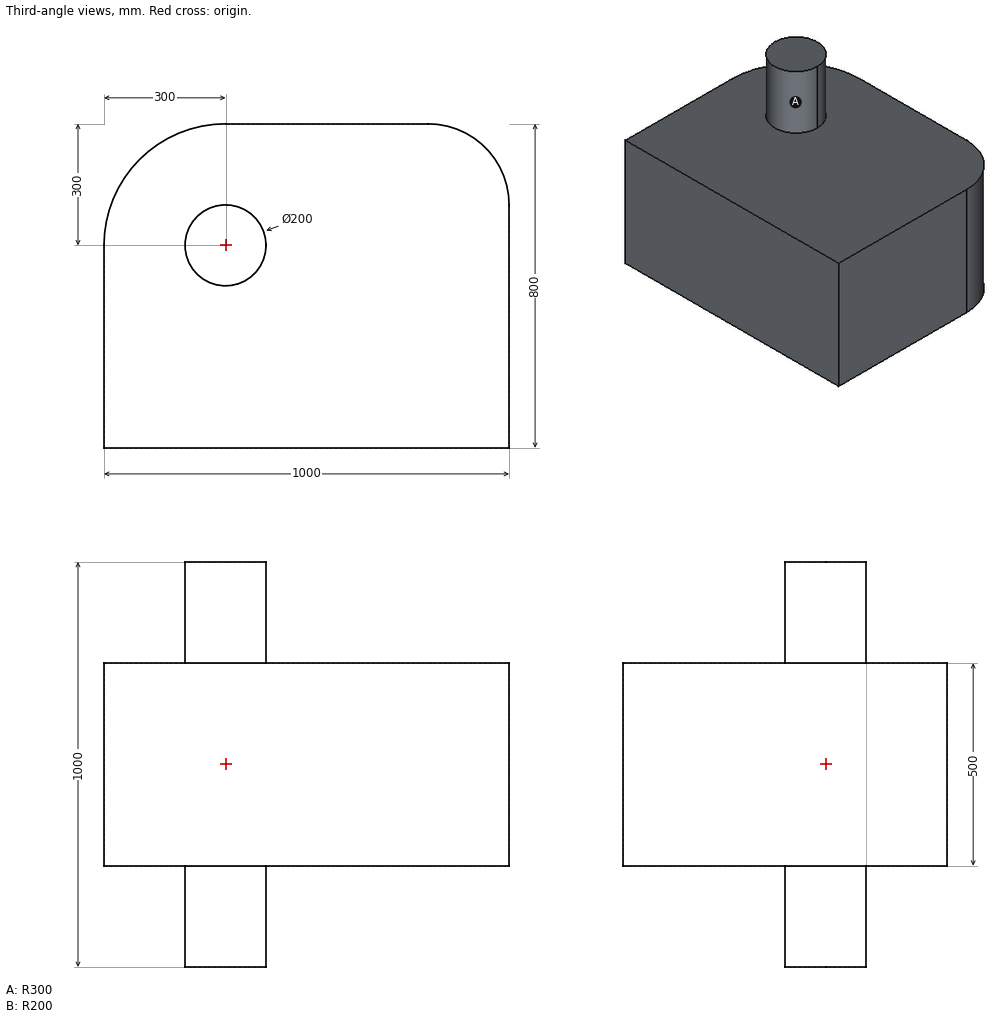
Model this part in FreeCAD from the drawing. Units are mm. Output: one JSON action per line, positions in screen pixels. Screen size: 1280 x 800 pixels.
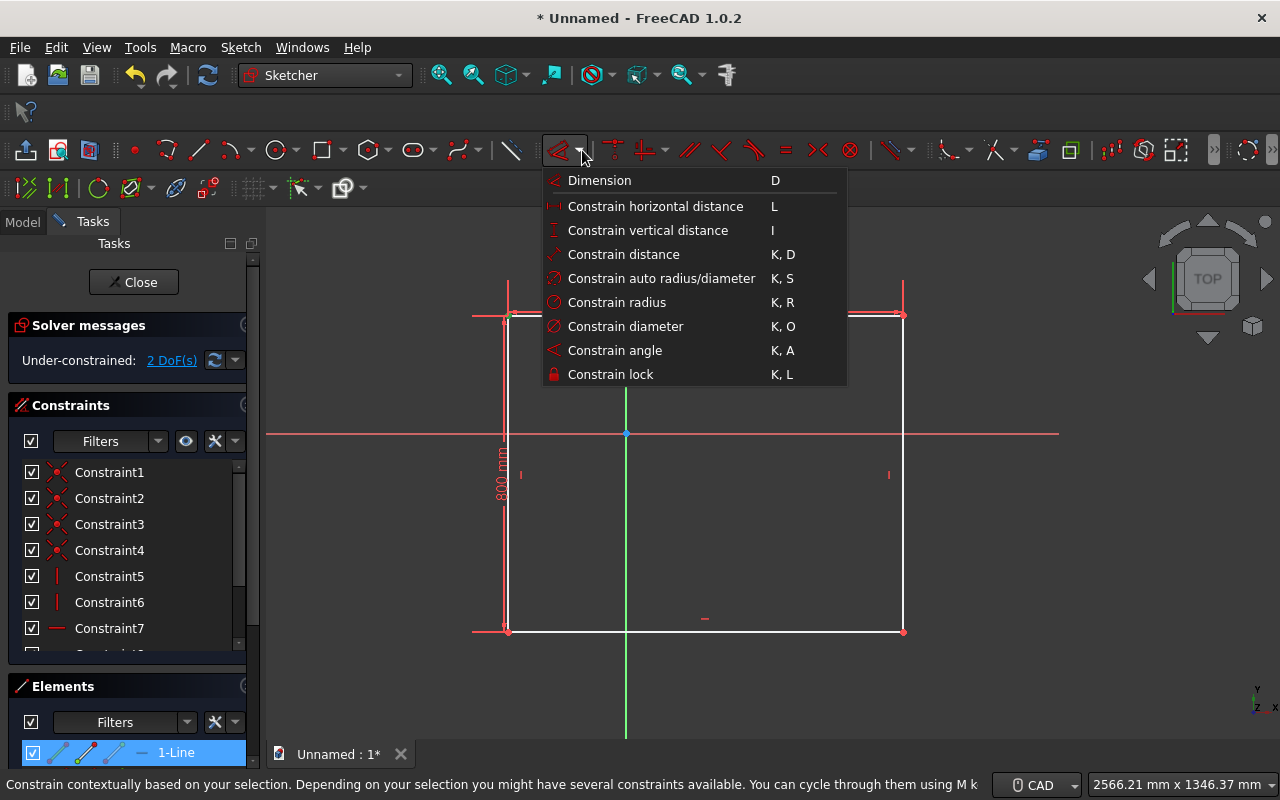
{"action": "left_click", "coordinate": [695, 206]}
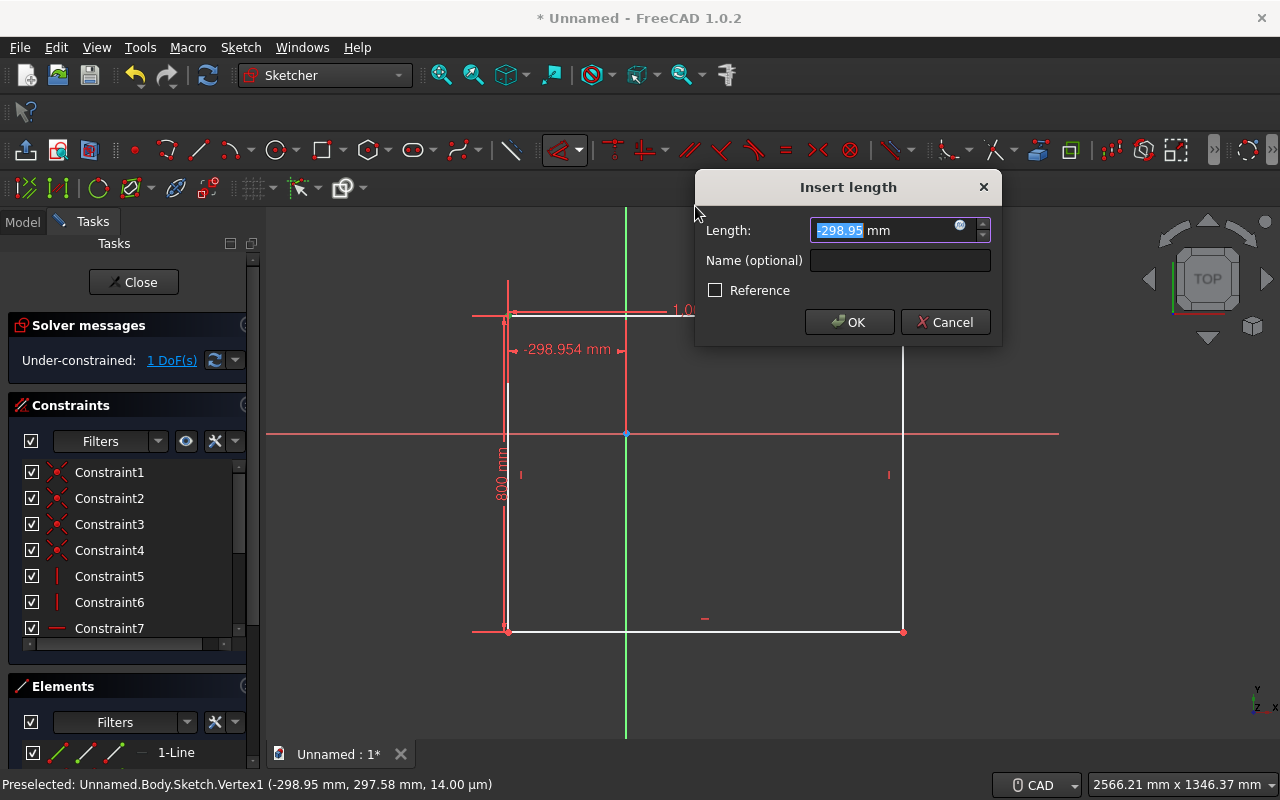
{"action": "type", "text": "-300"}
{"action": "key", "text": "Return"}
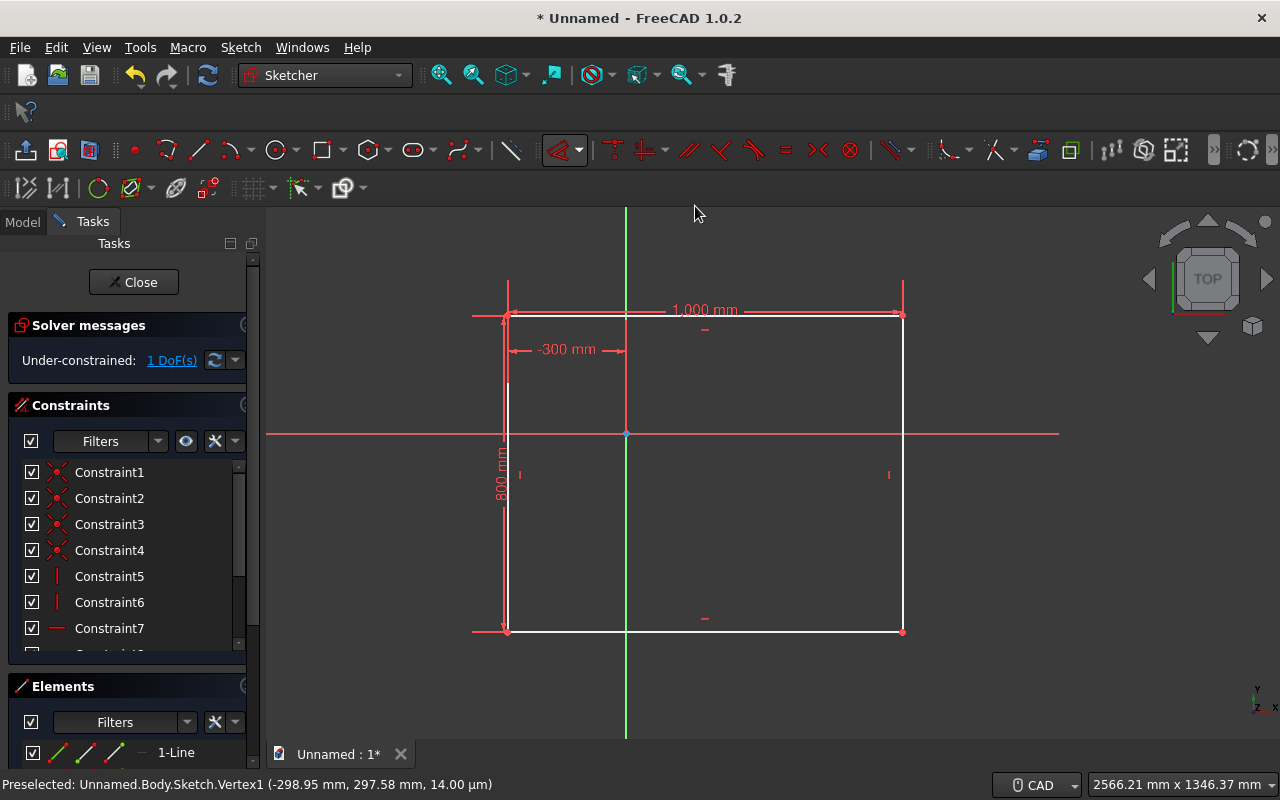
{"action": "left_click", "coordinate": [508, 316]}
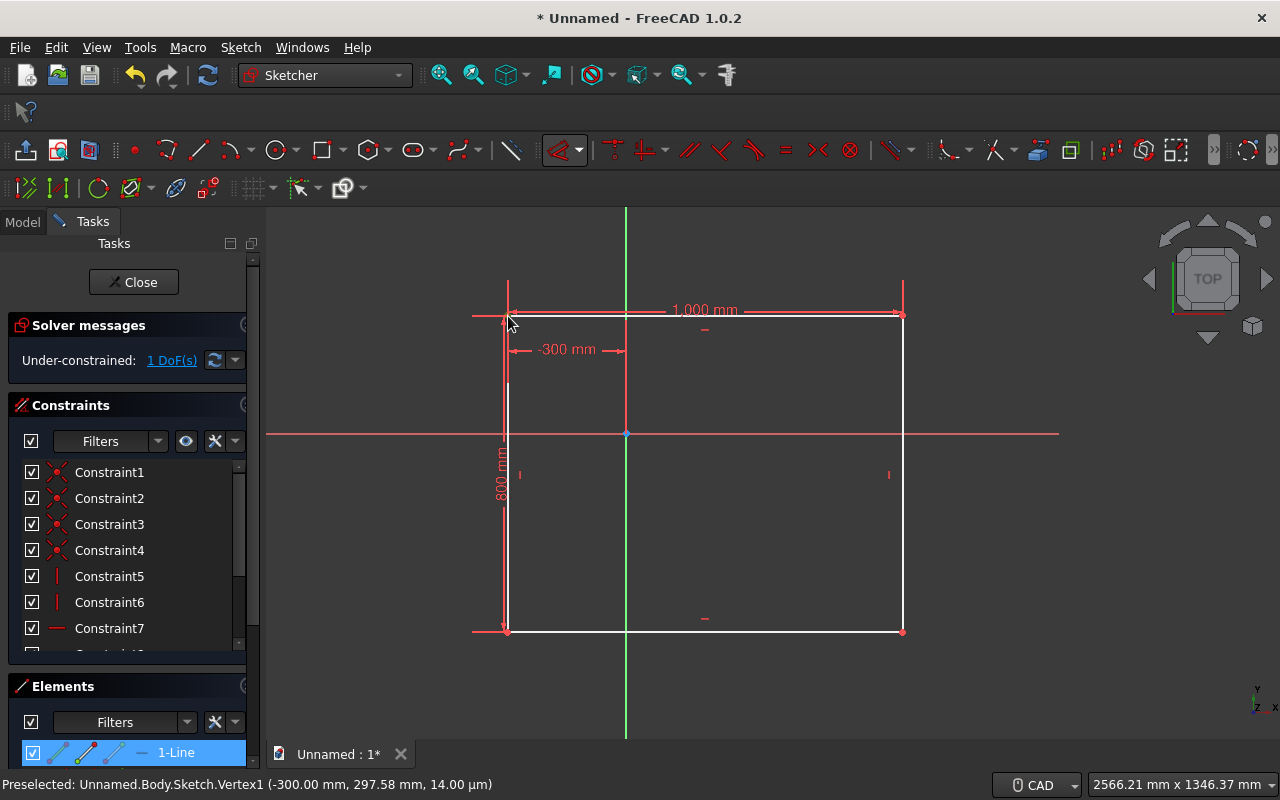
{"action": "key", "text": "i"}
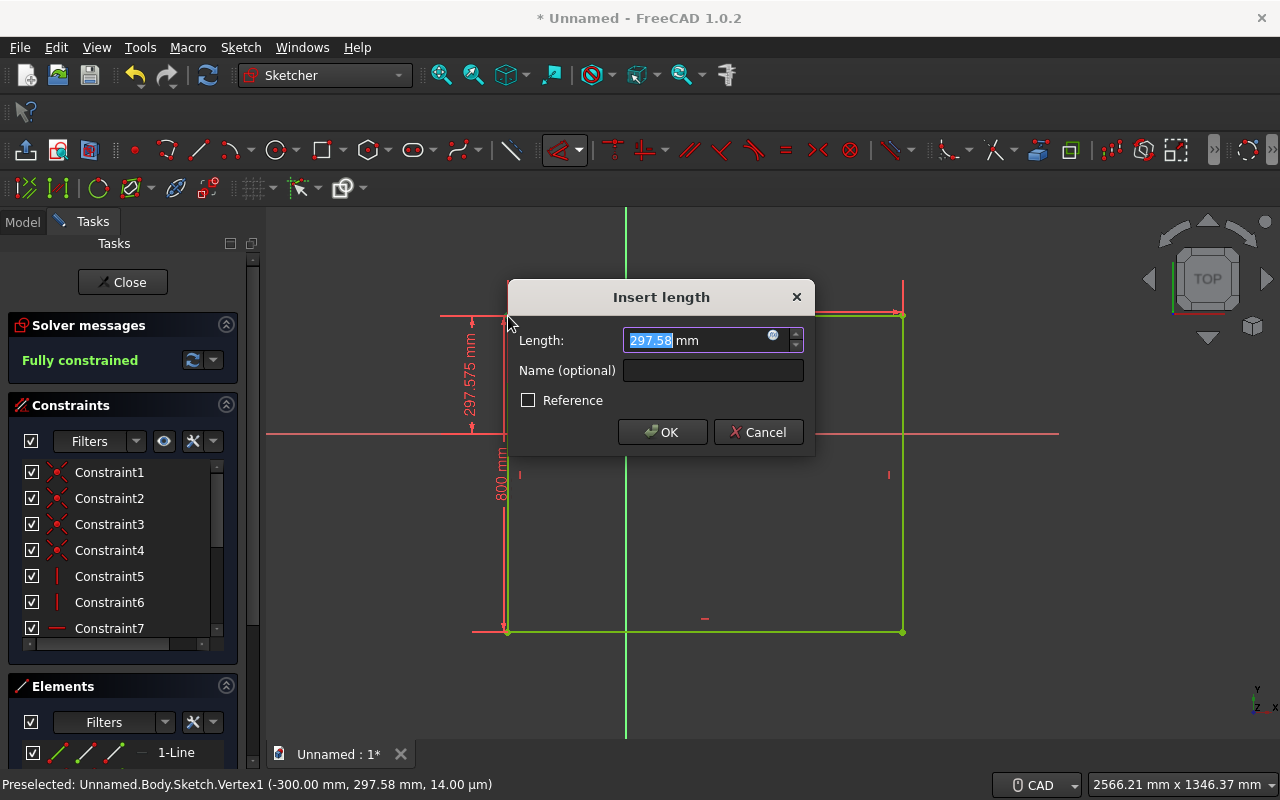
{"action": "type", "text": "300"}
{"action": "key", "text": "Return"}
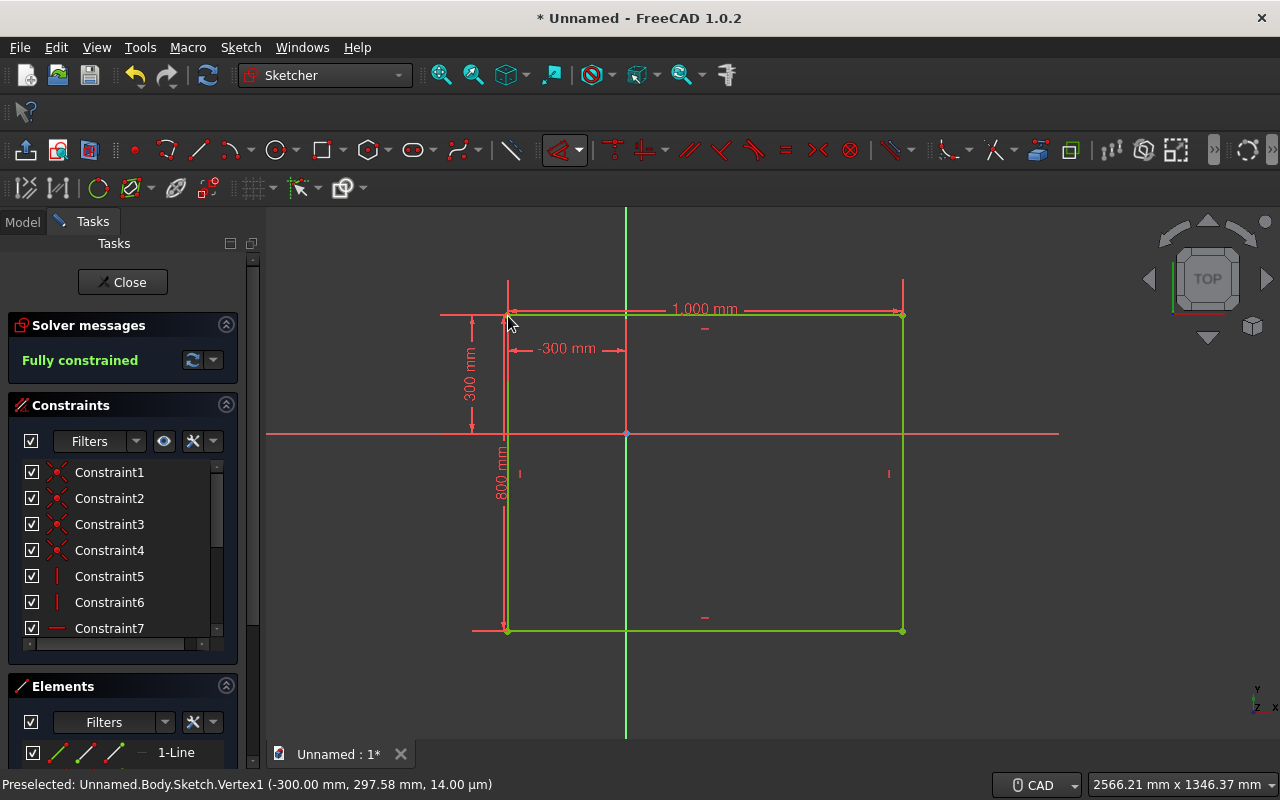
{"action": "left_click", "coordinate": [123, 282]}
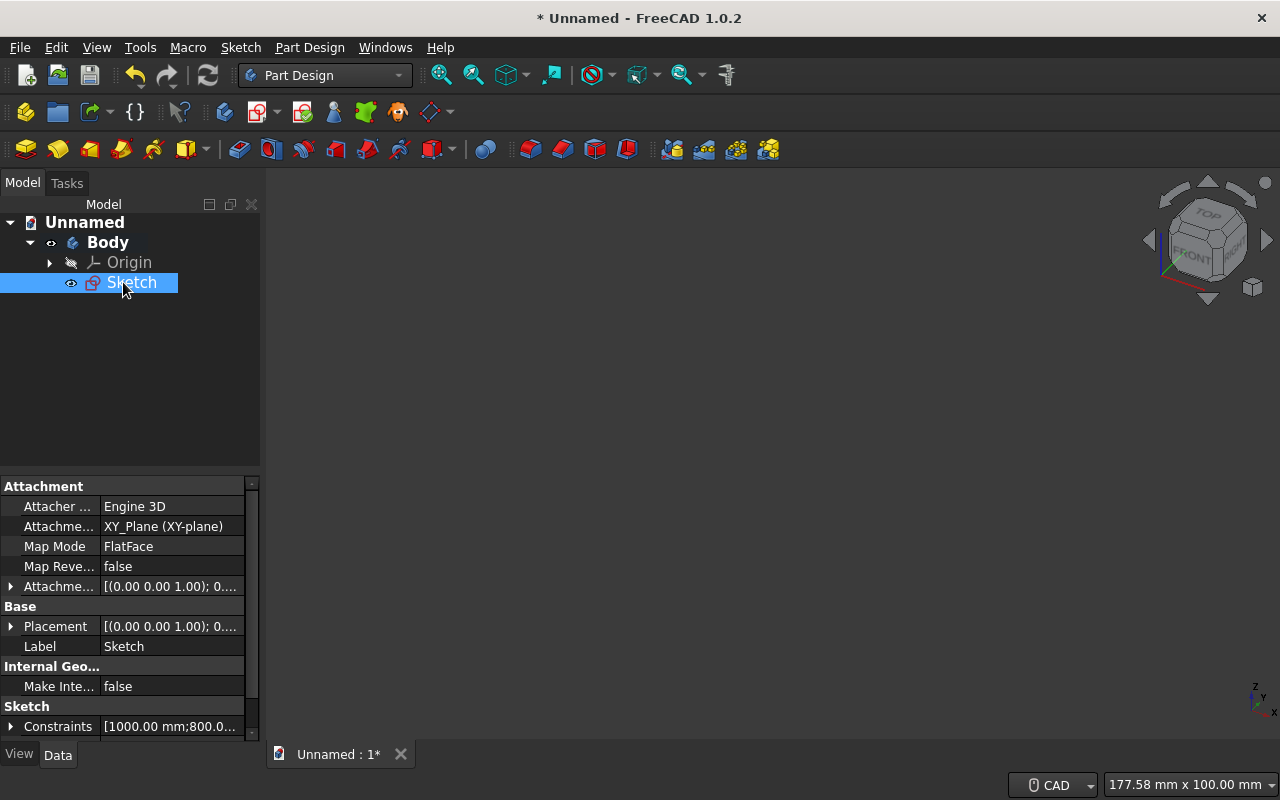
{"action": "left_click", "coordinate": [26, 150]}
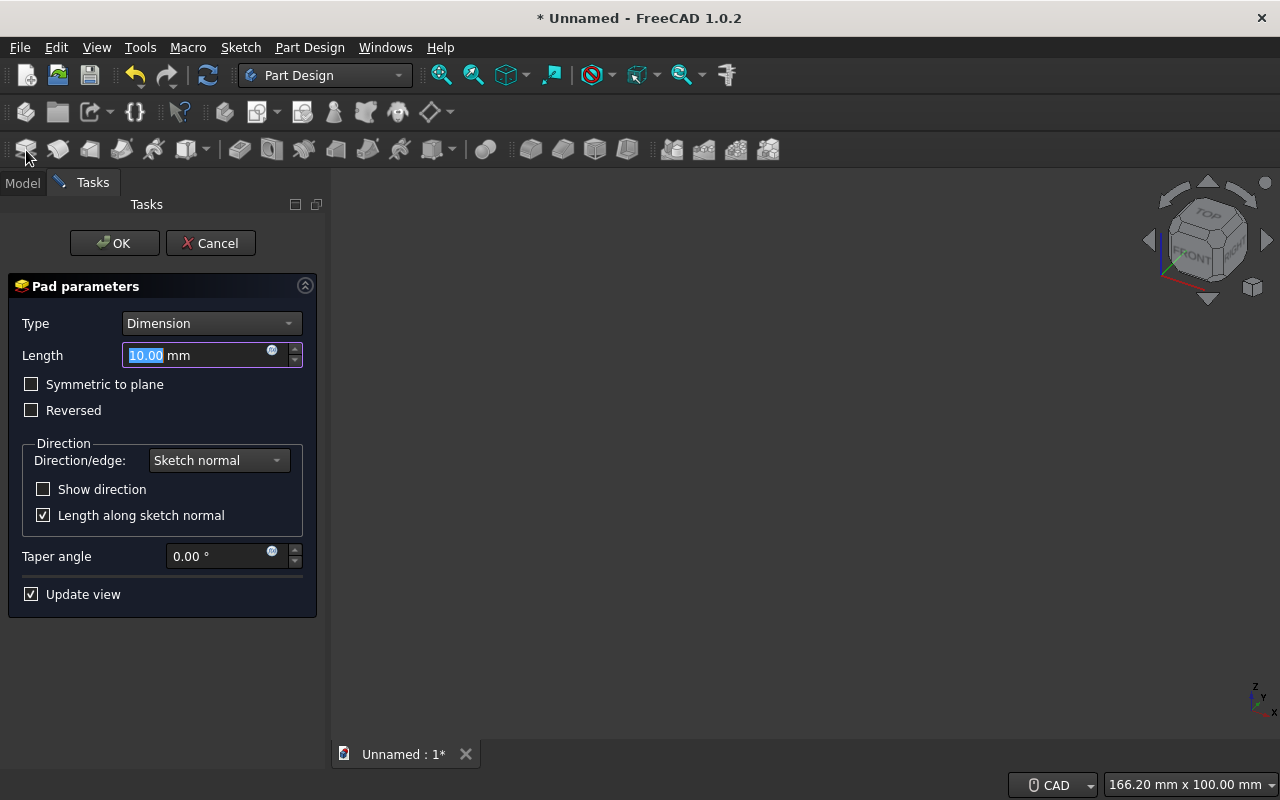
{"action": "type", "text": "500"}
{"action": "key", "text": "Tab"}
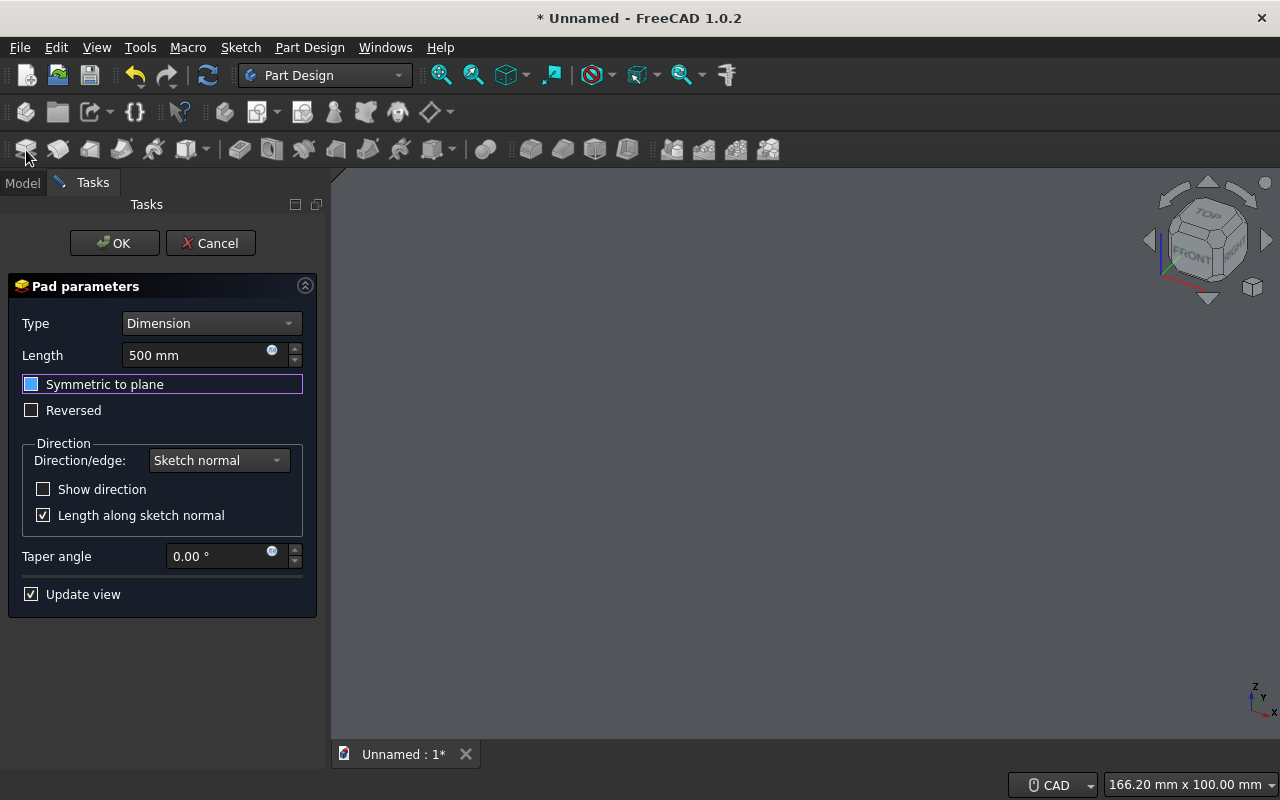
{"action": "left_click", "coordinate": [30, 384]}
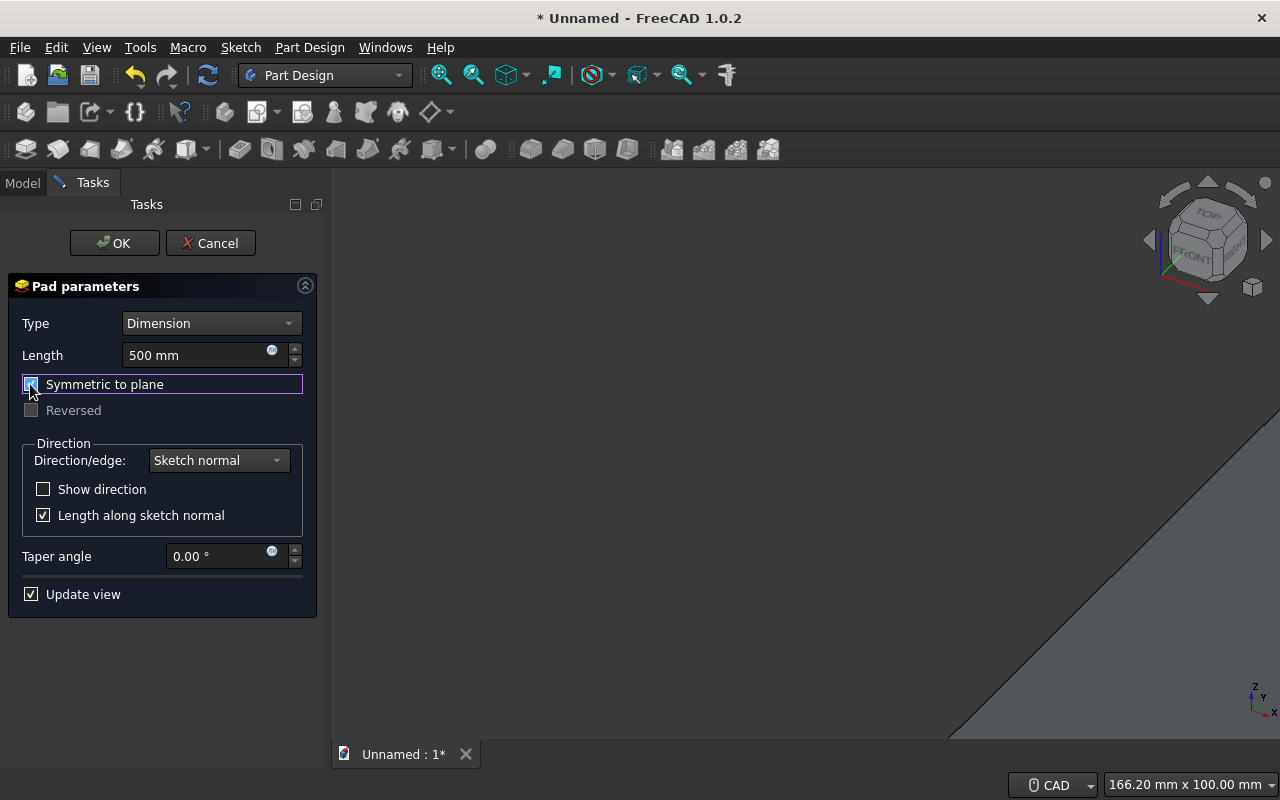
{"action": "left_click", "coordinate": [115, 243]}